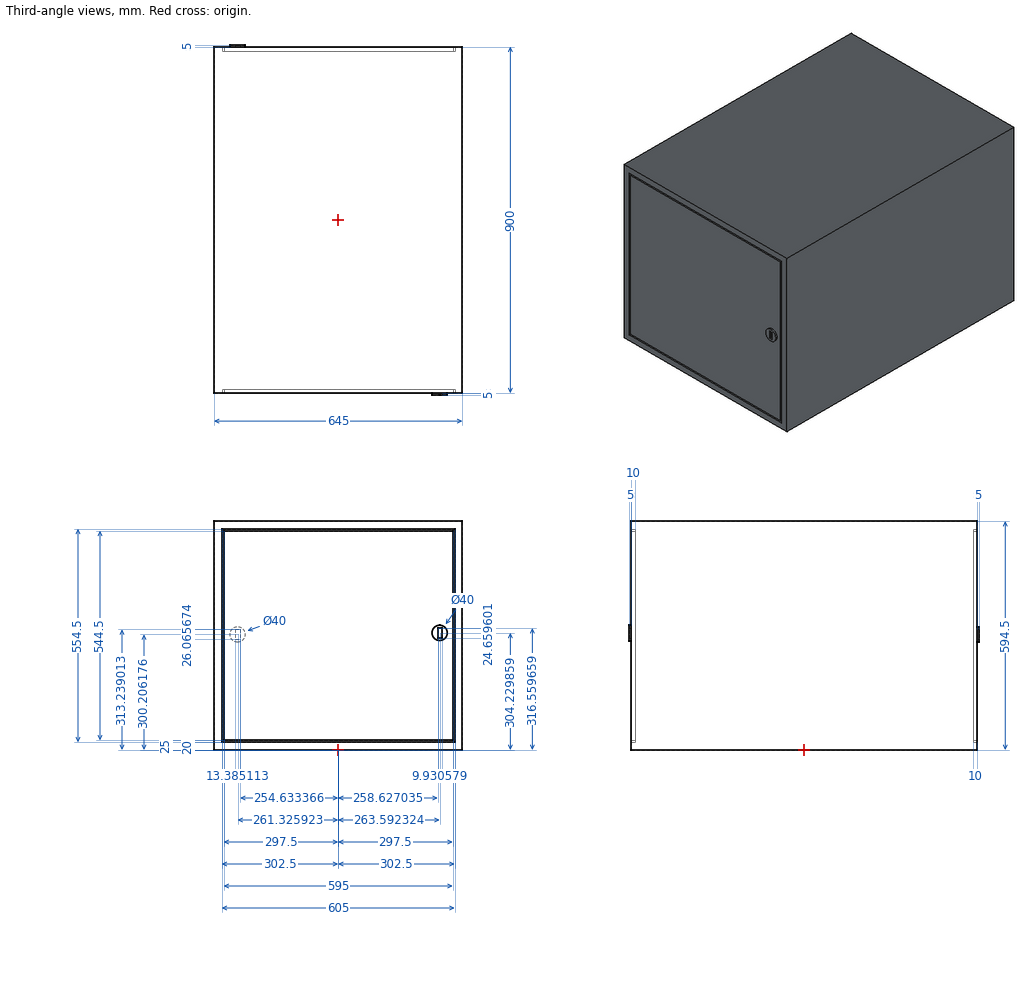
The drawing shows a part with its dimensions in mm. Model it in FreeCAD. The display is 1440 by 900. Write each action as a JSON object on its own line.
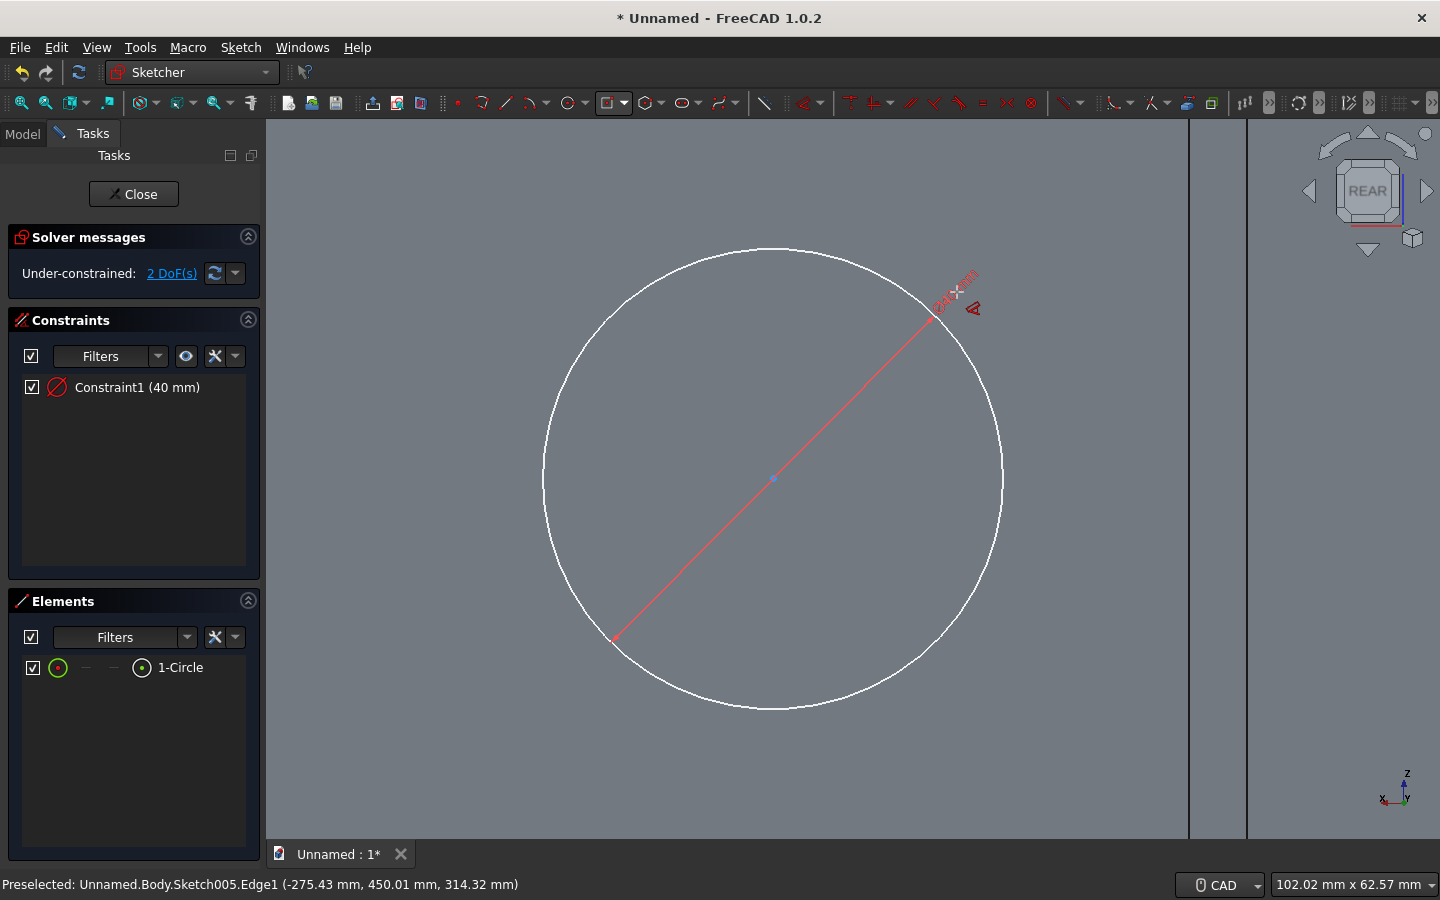
{"action": "left_click", "coordinate": [773, 479]}
{"action": "left_click", "coordinate": [423, 445]}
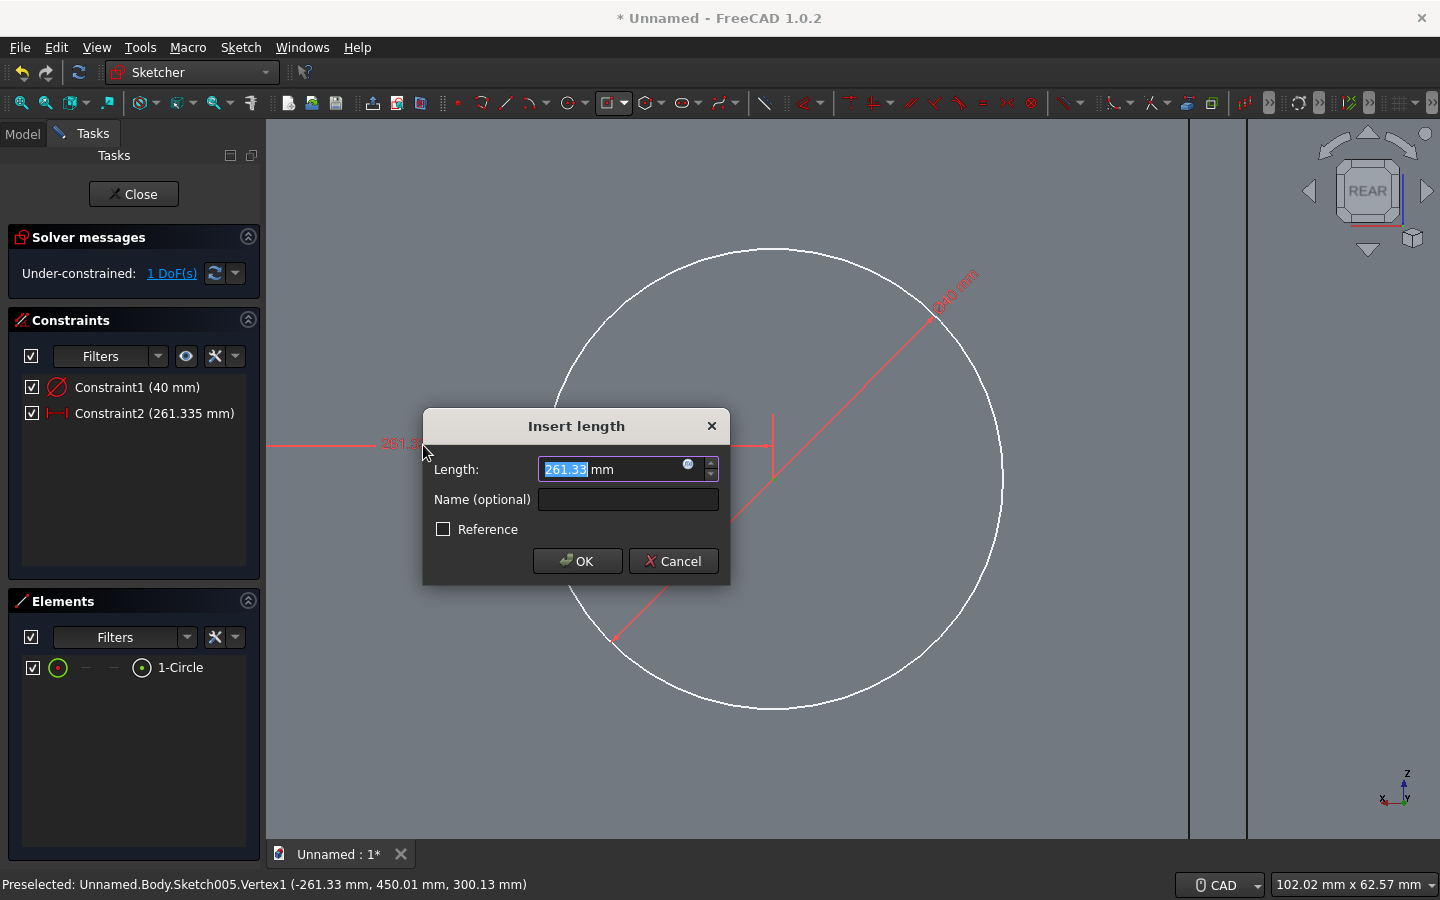
{"action": "type", "text": "261.325923"}
{"action": "key", "text": "Return"}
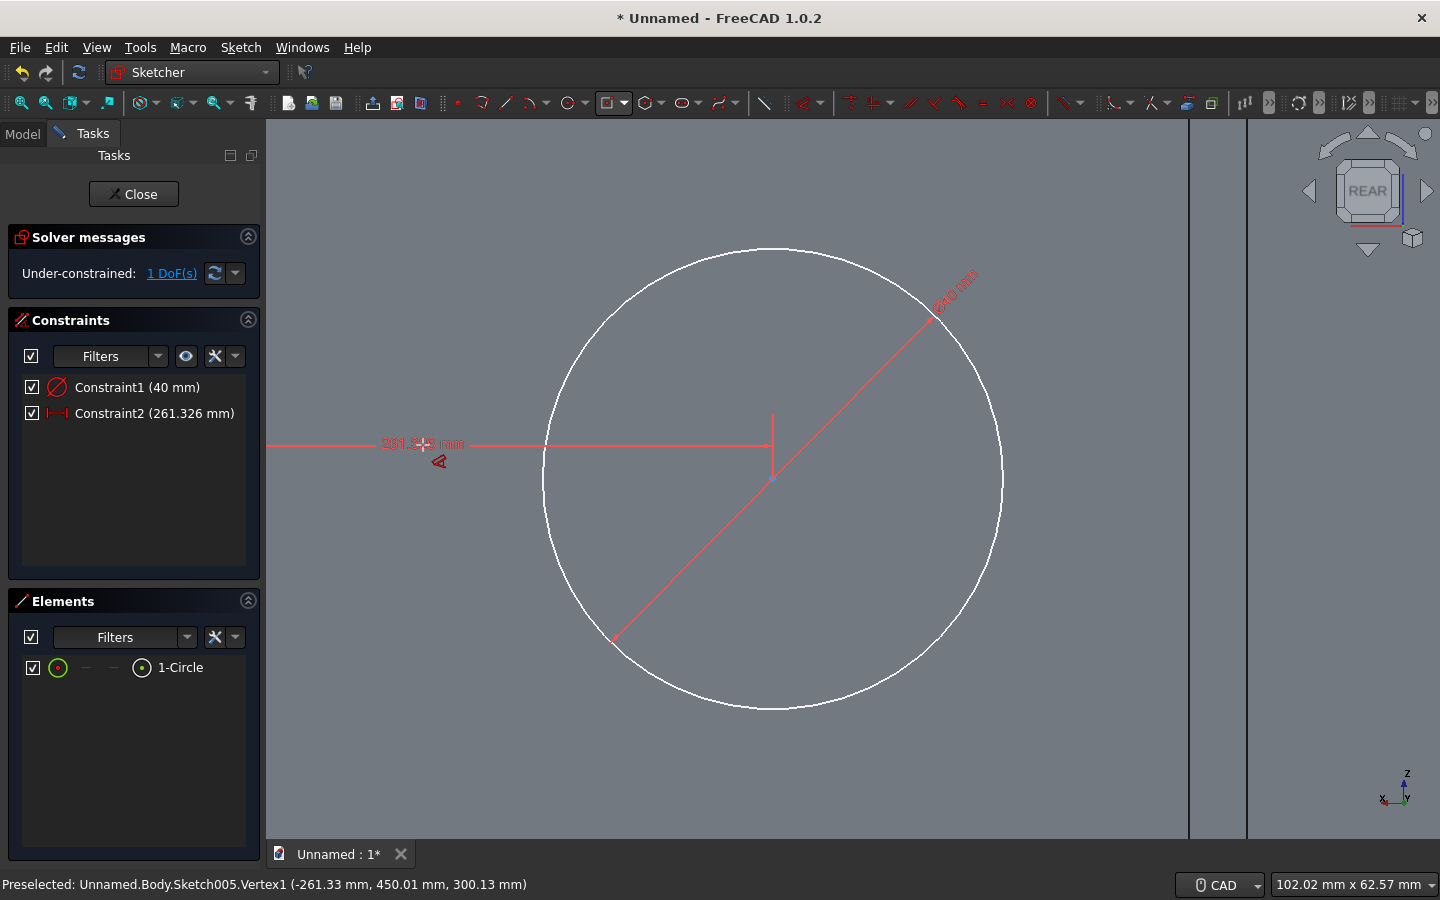
{"action": "left_click", "coordinate": [773, 479]}
{"action": "left_click", "coordinate": [807, 645]}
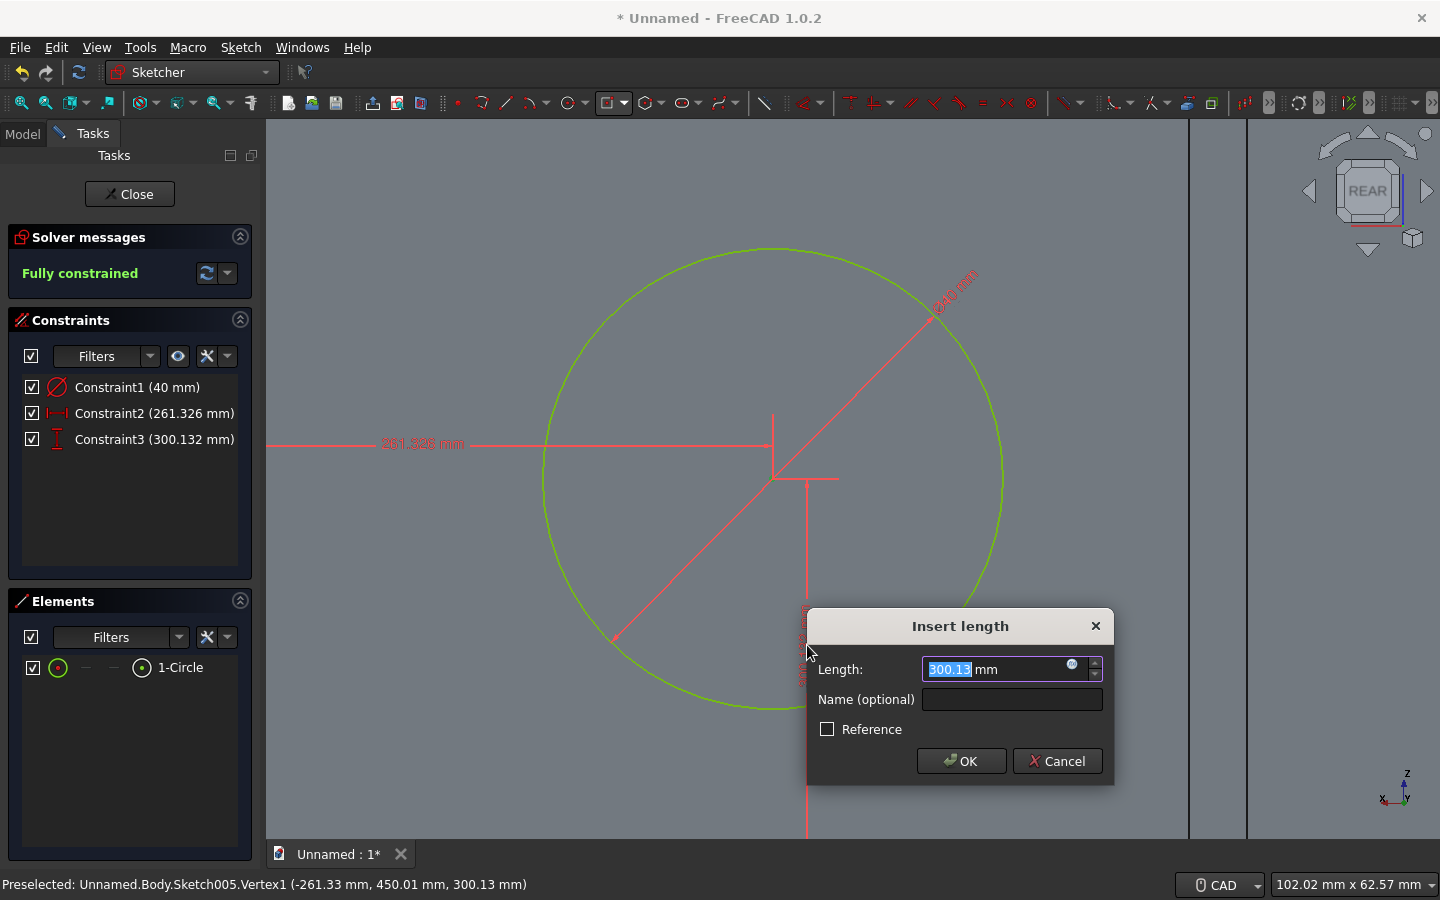
{"action": "type", "text": "300.206176"}
{"action": "key", "text": "Return"}
{"action": "key", "text": "Escape"}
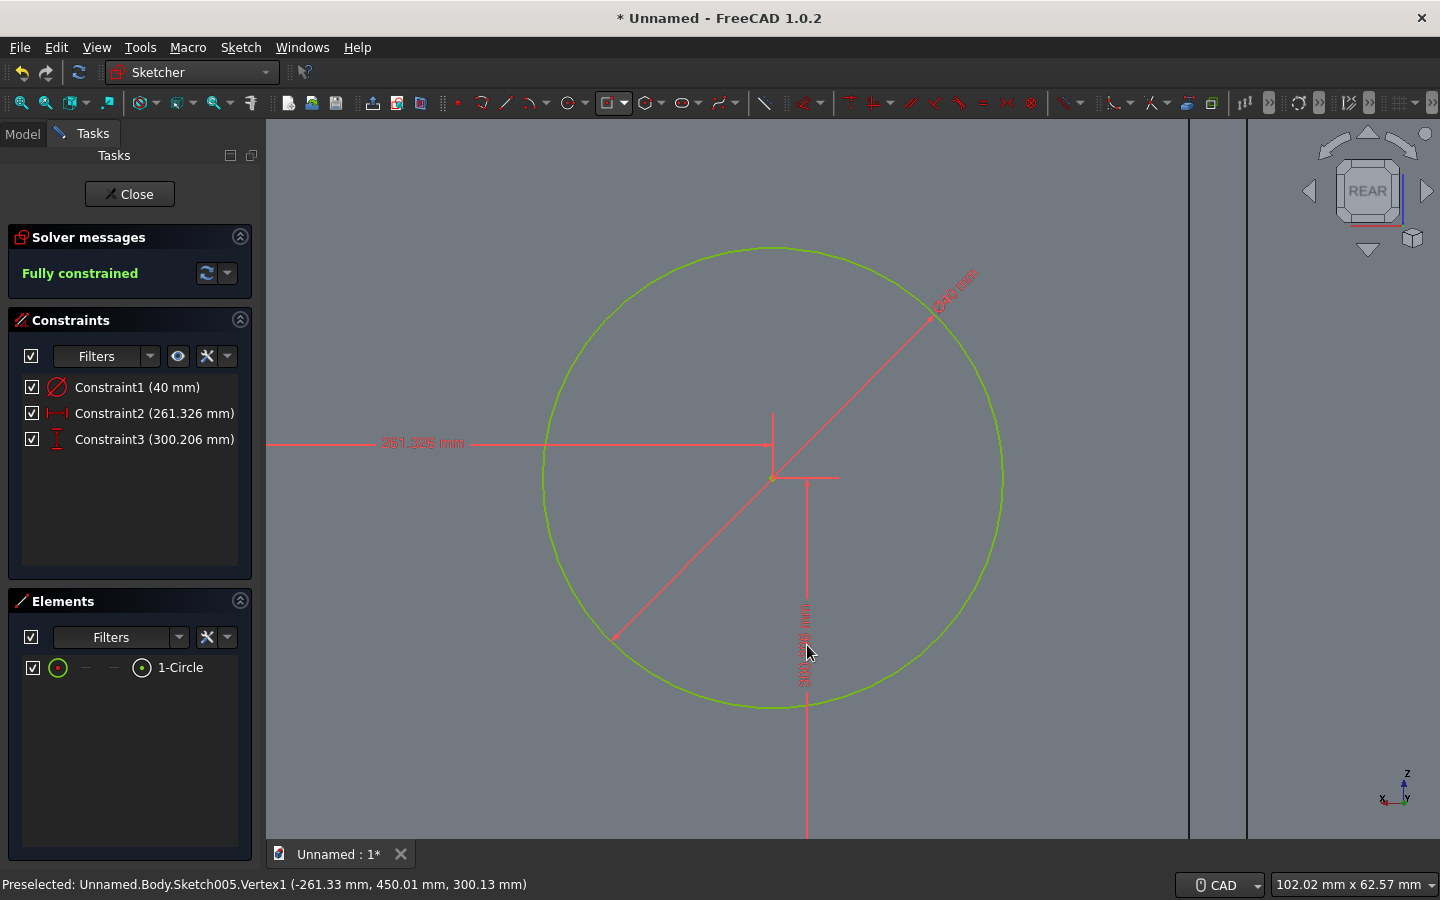
{"action": "left_click", "coordinate": [130, 194]}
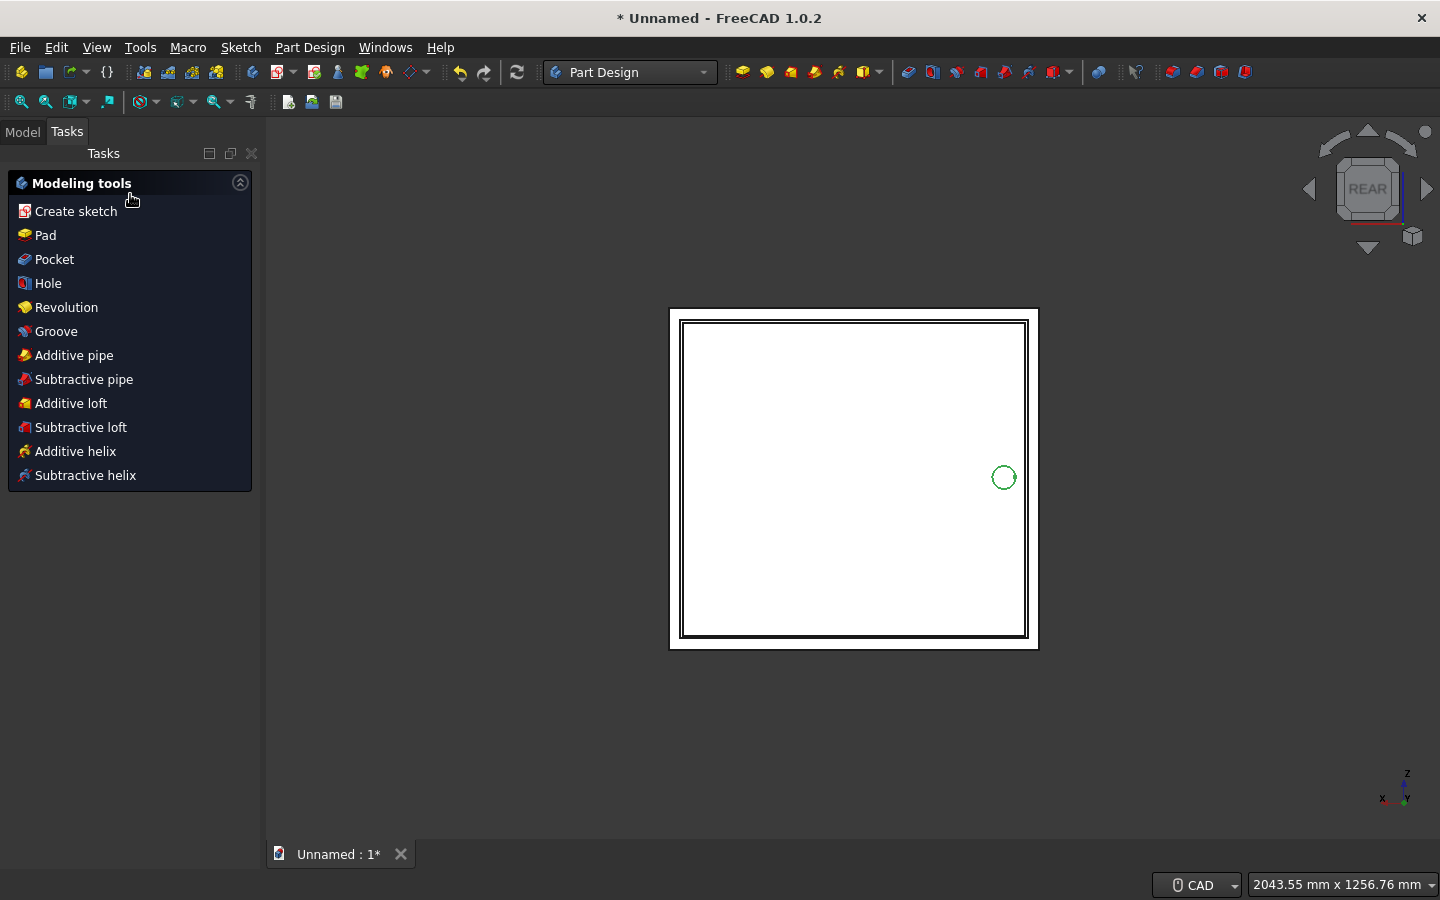
{"action": "left_click", "coordinate": [744, 72]}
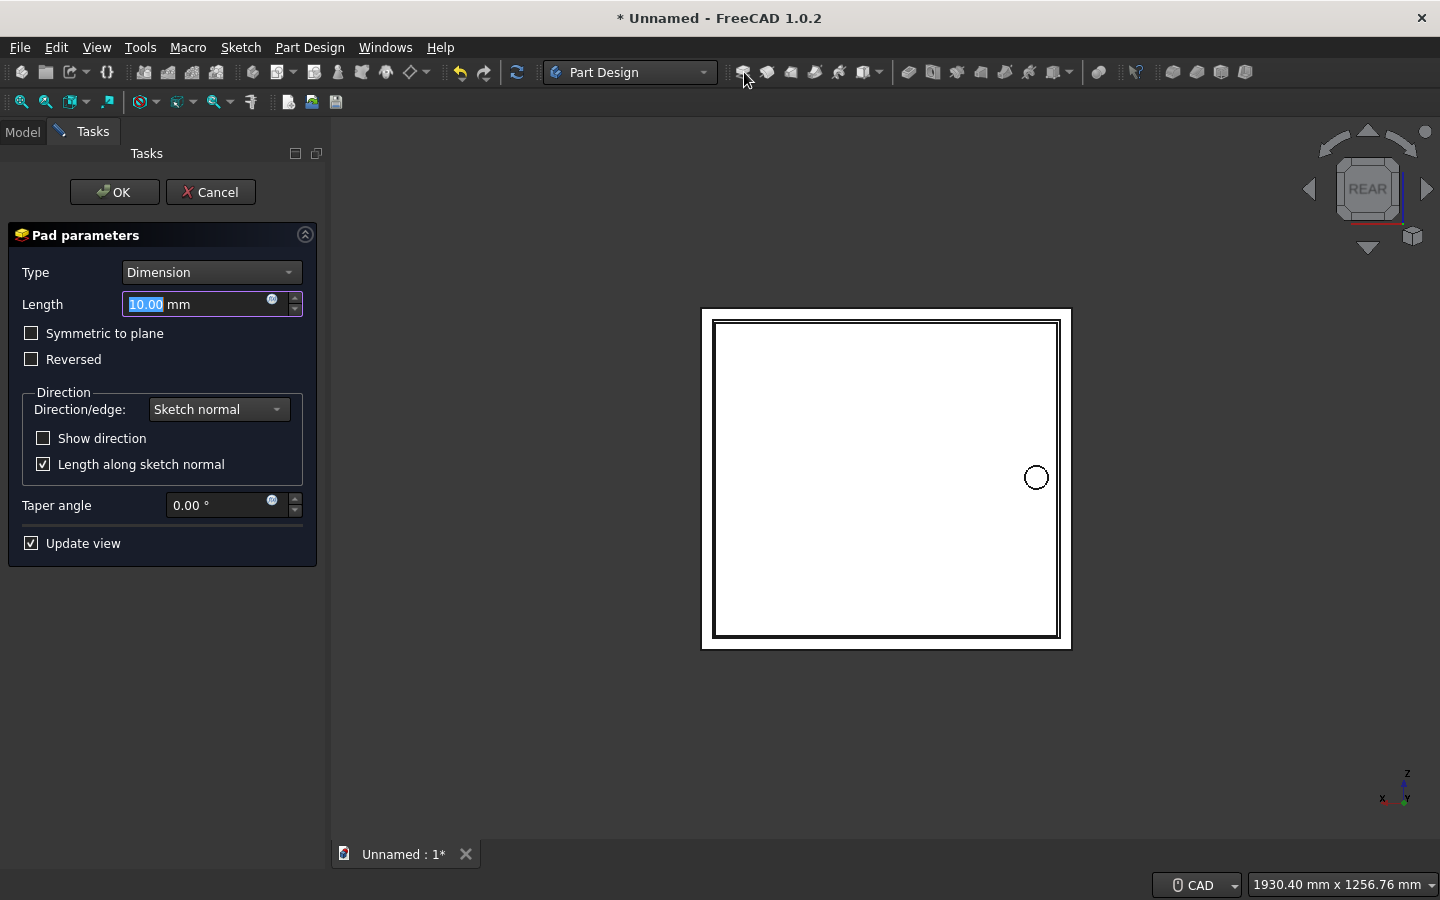
{"action": "type", "text": "5"}
{"action": "key", "text": "Tab"}